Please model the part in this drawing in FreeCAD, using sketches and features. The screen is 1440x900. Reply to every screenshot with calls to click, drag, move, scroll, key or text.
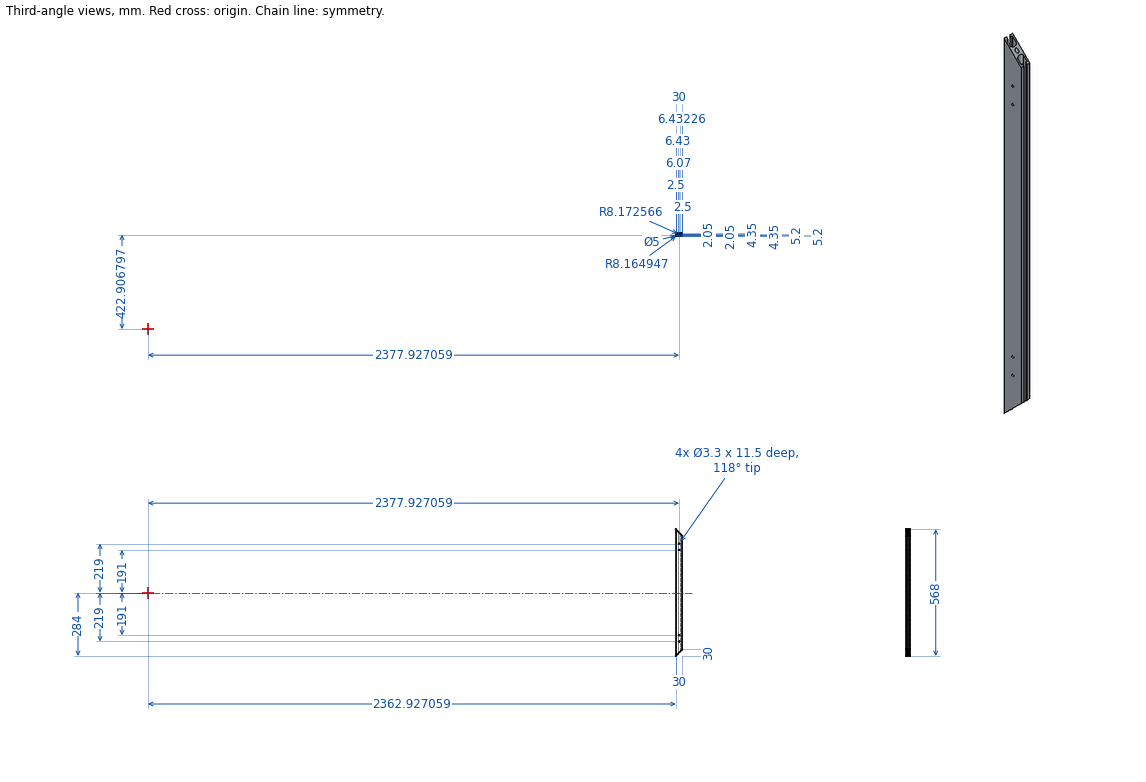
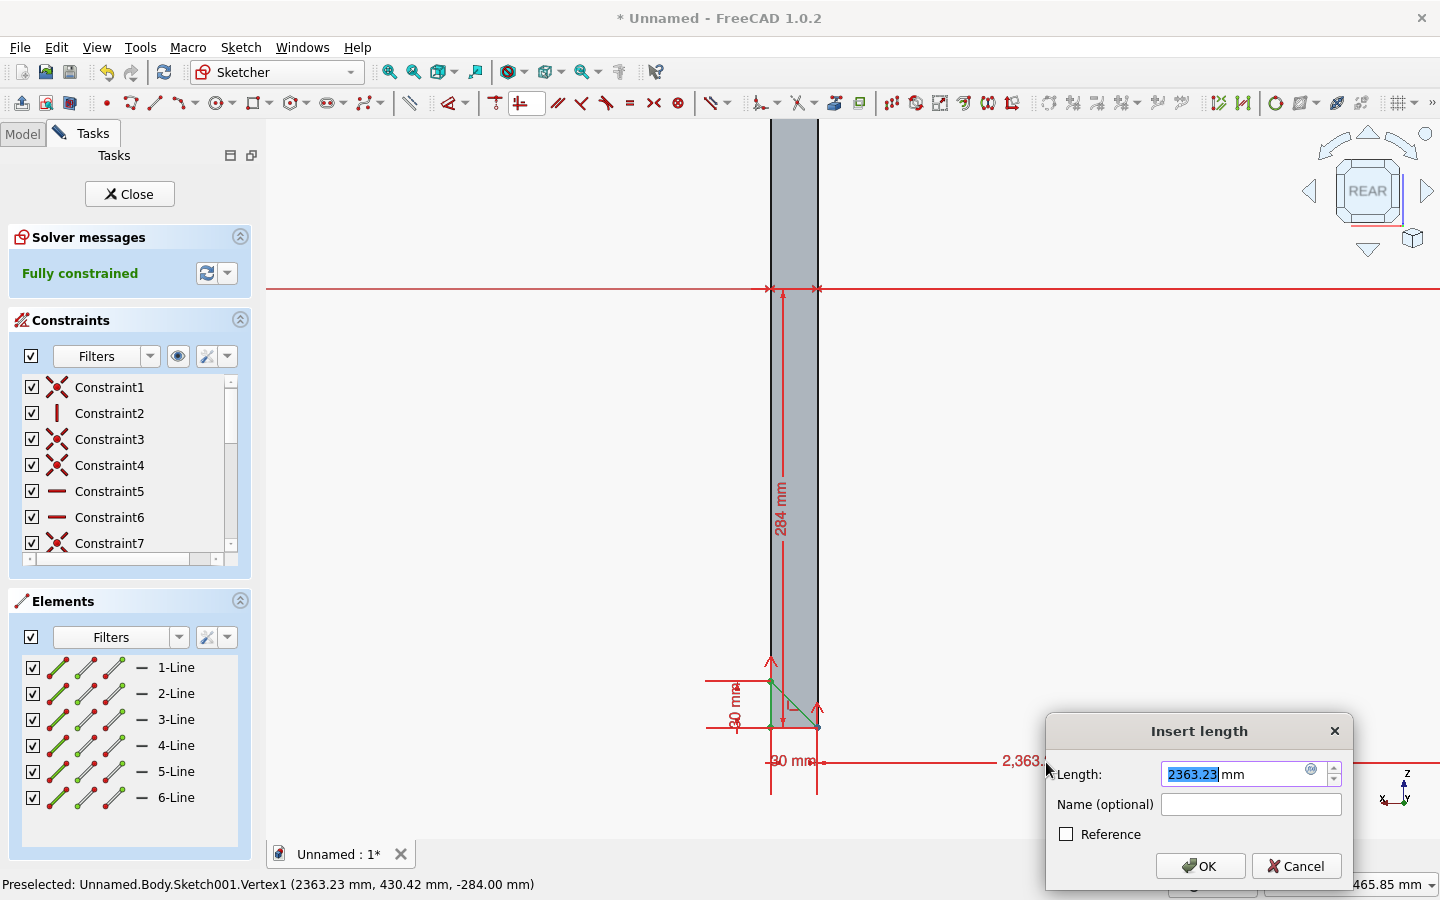
text(2362.927059)
key(Return)
key(Escape)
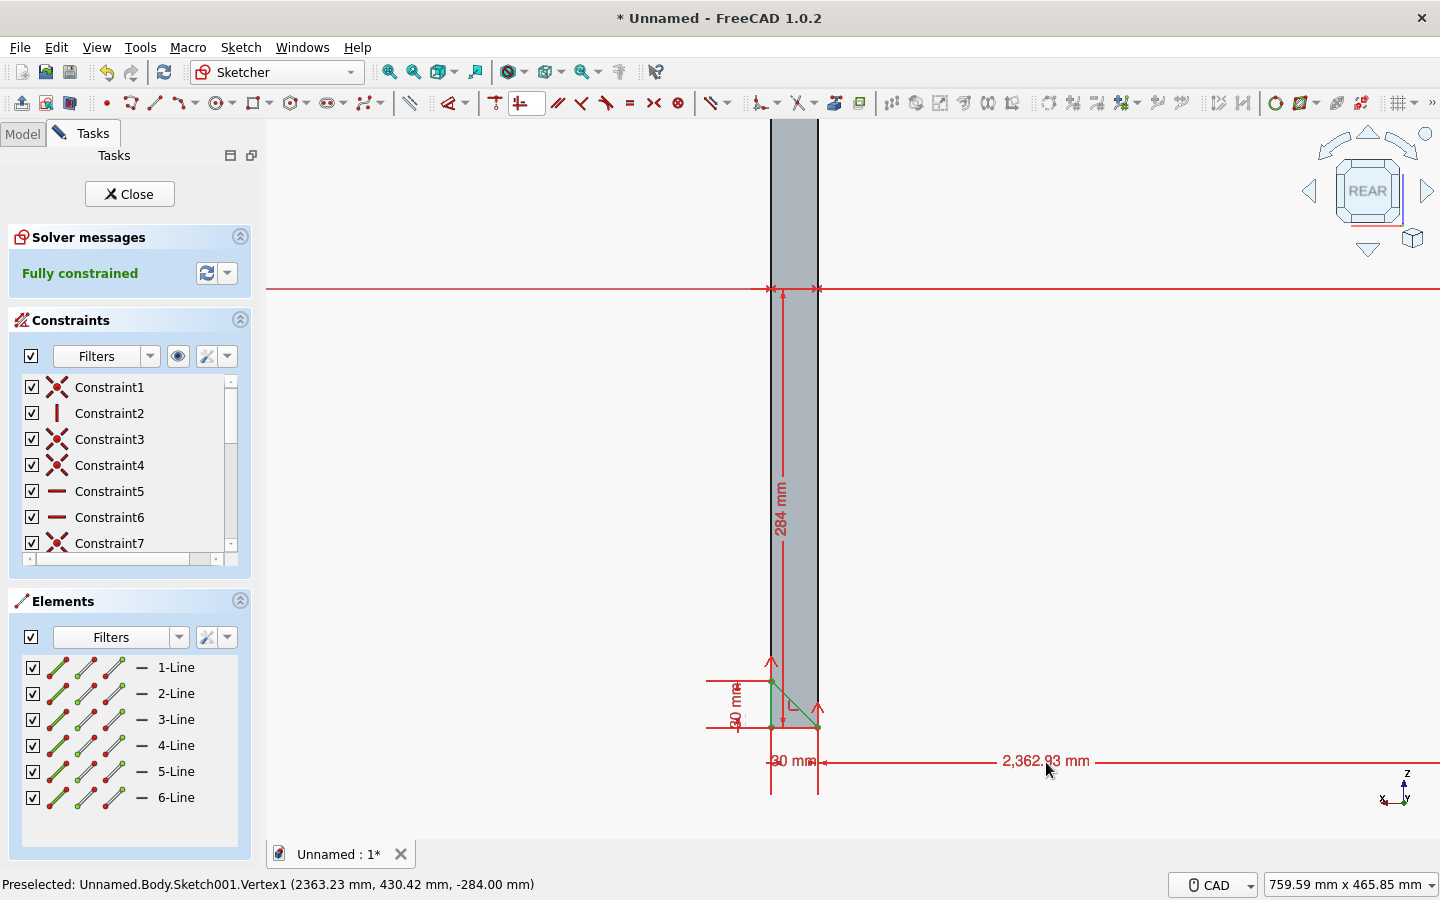
click(130, 194)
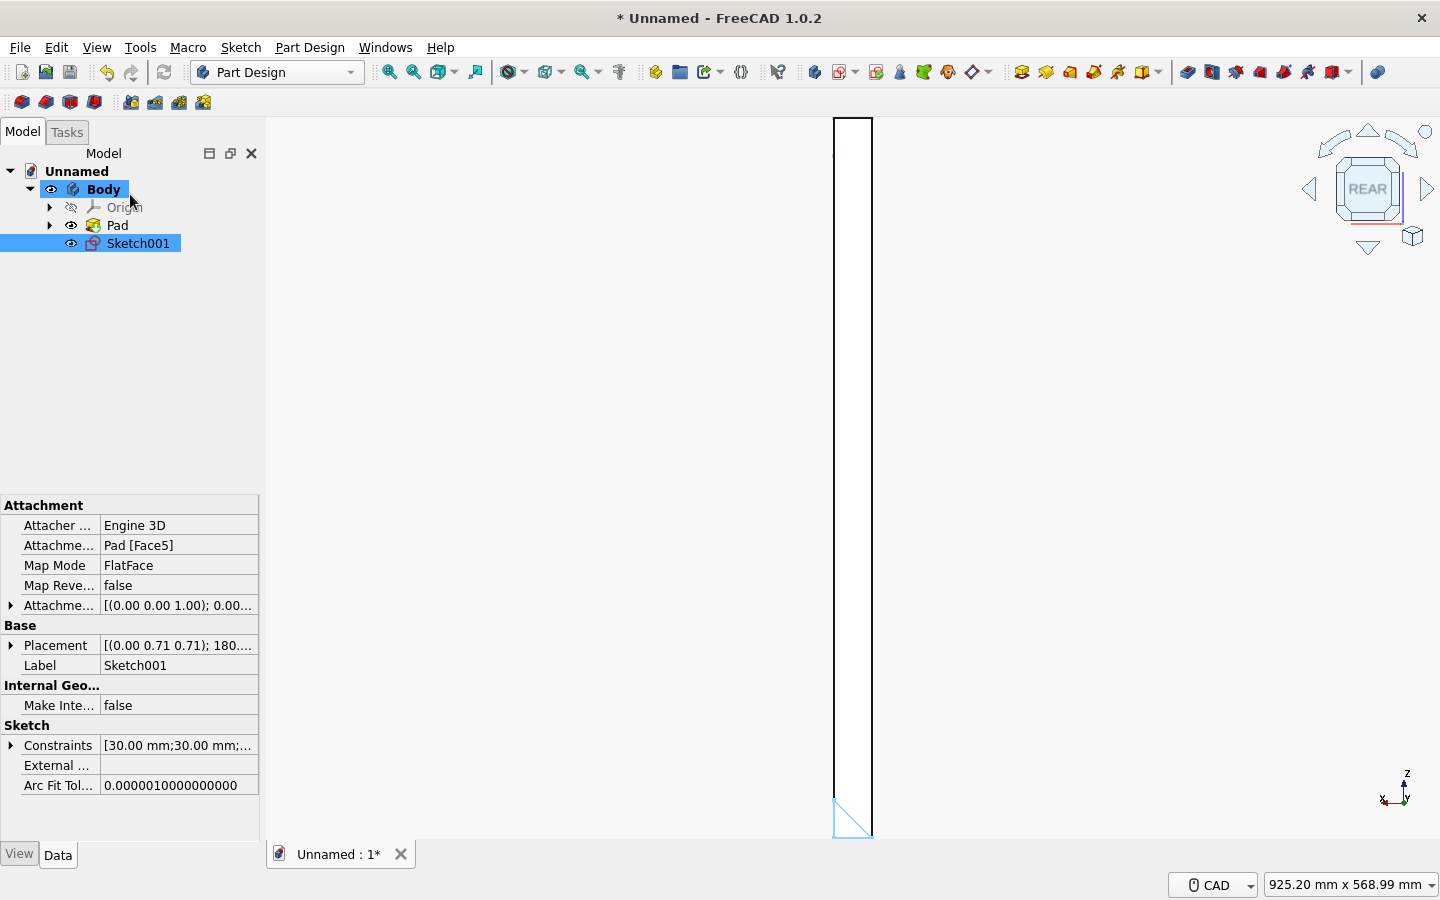
click(1188, 72)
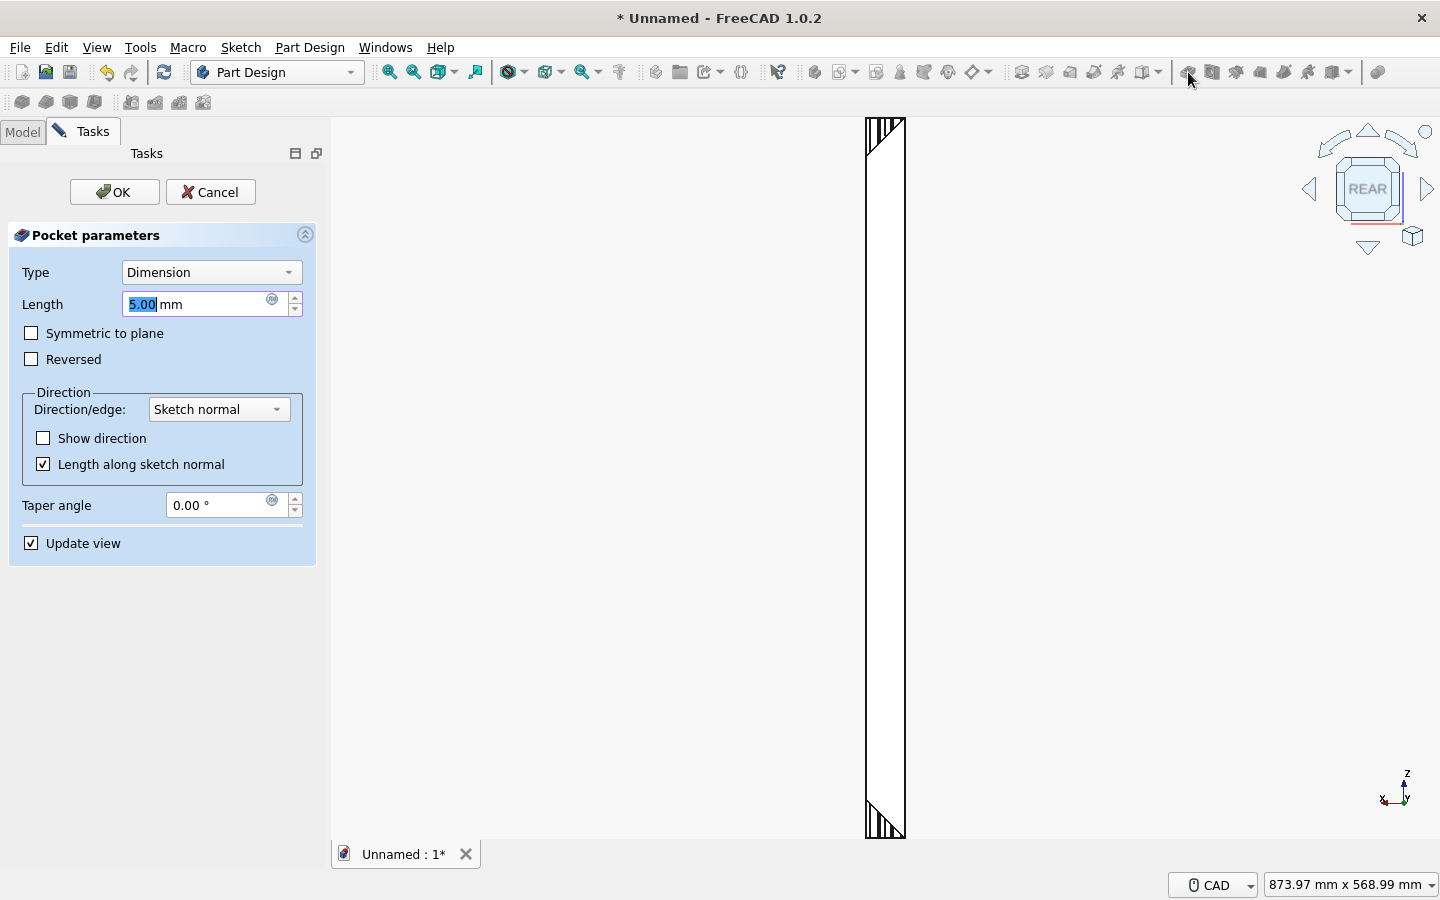
click(212, 272)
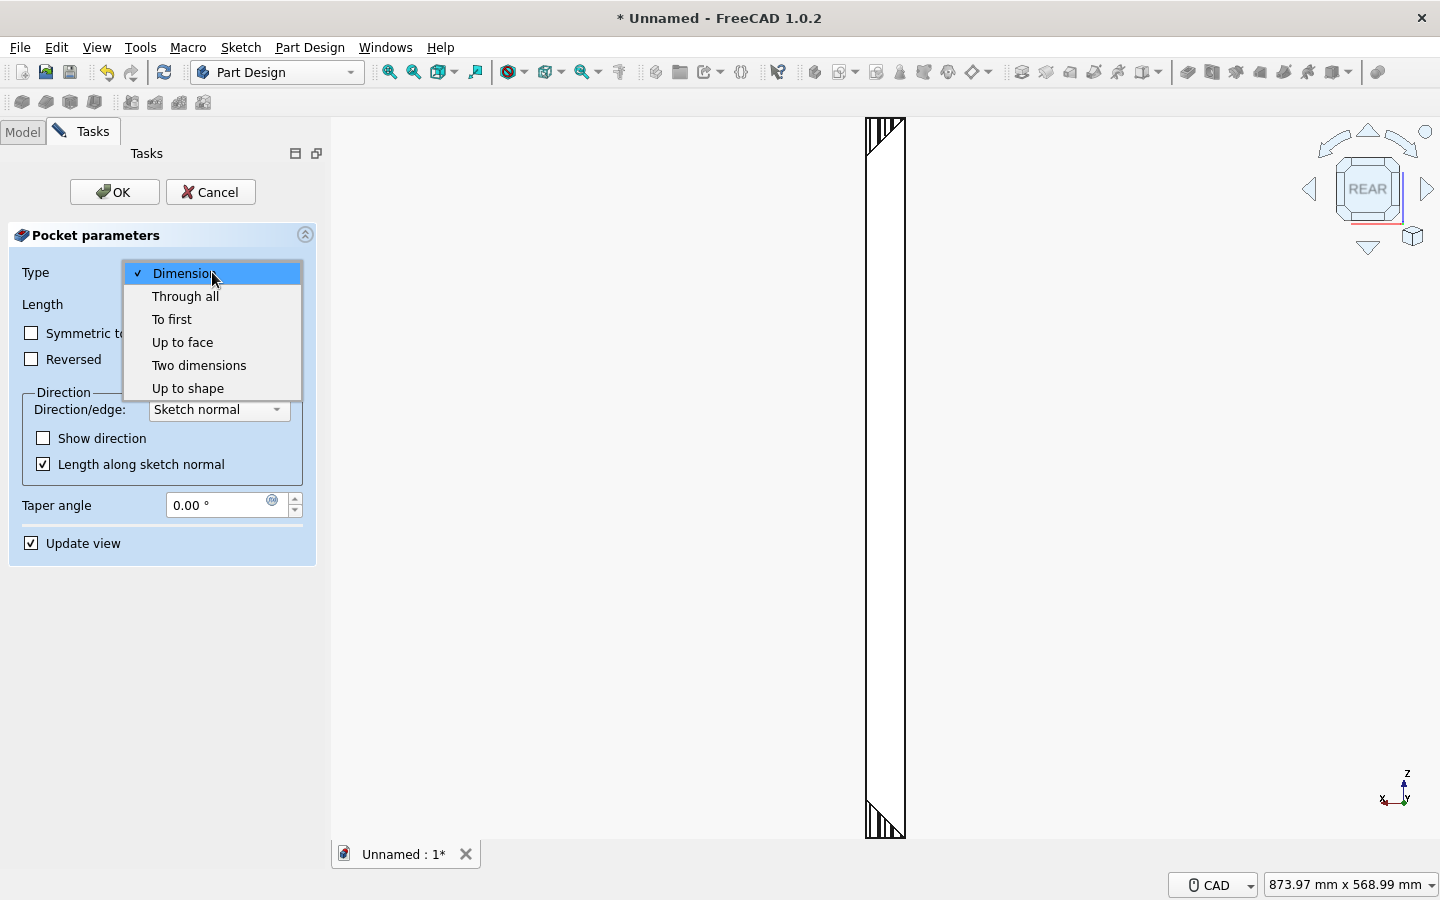
click(212, 296)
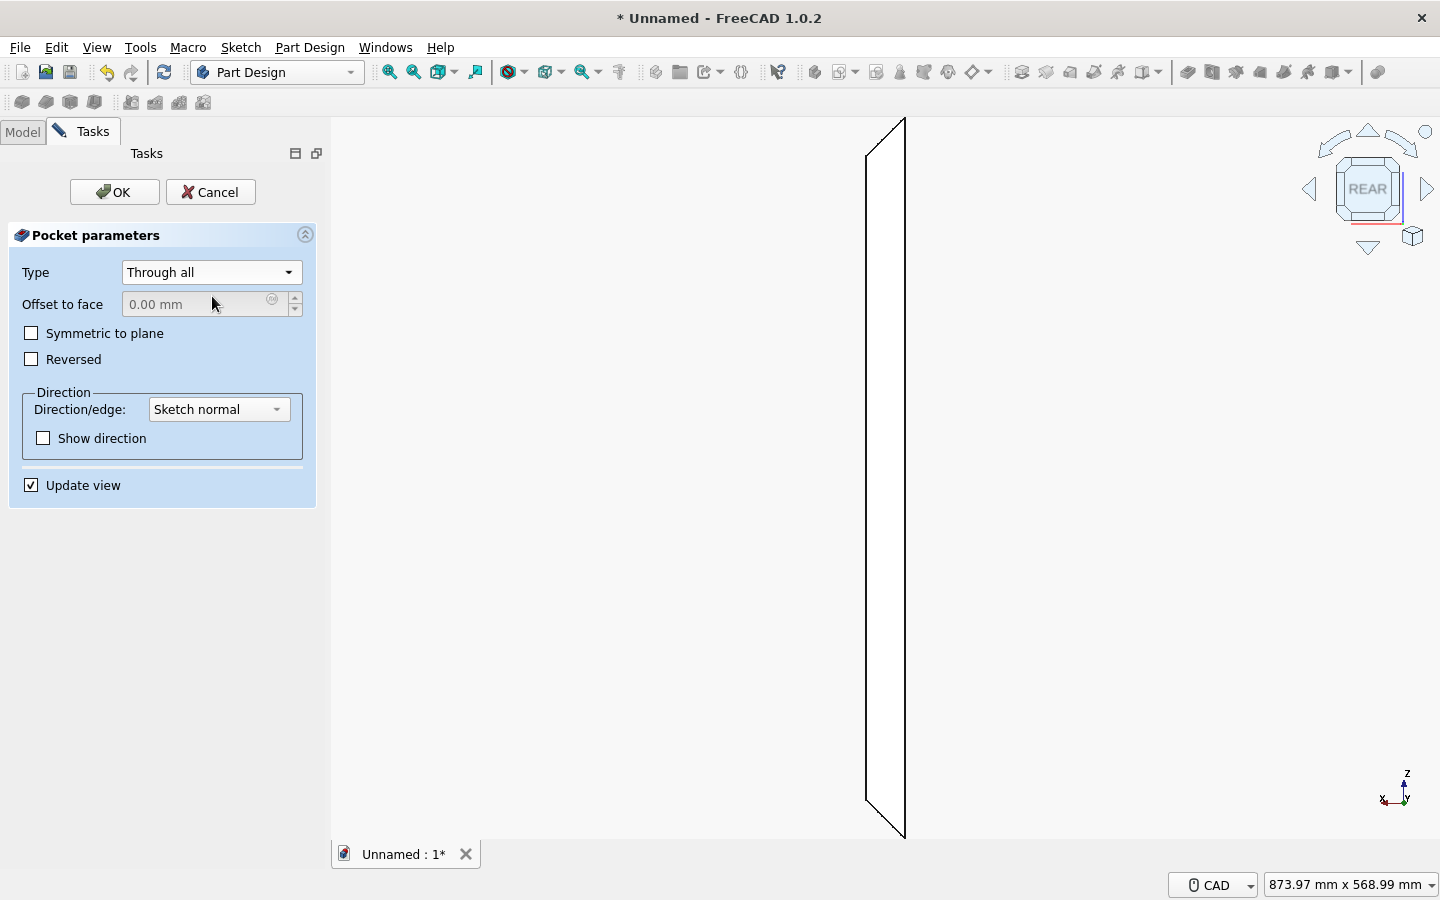
click(115, 192)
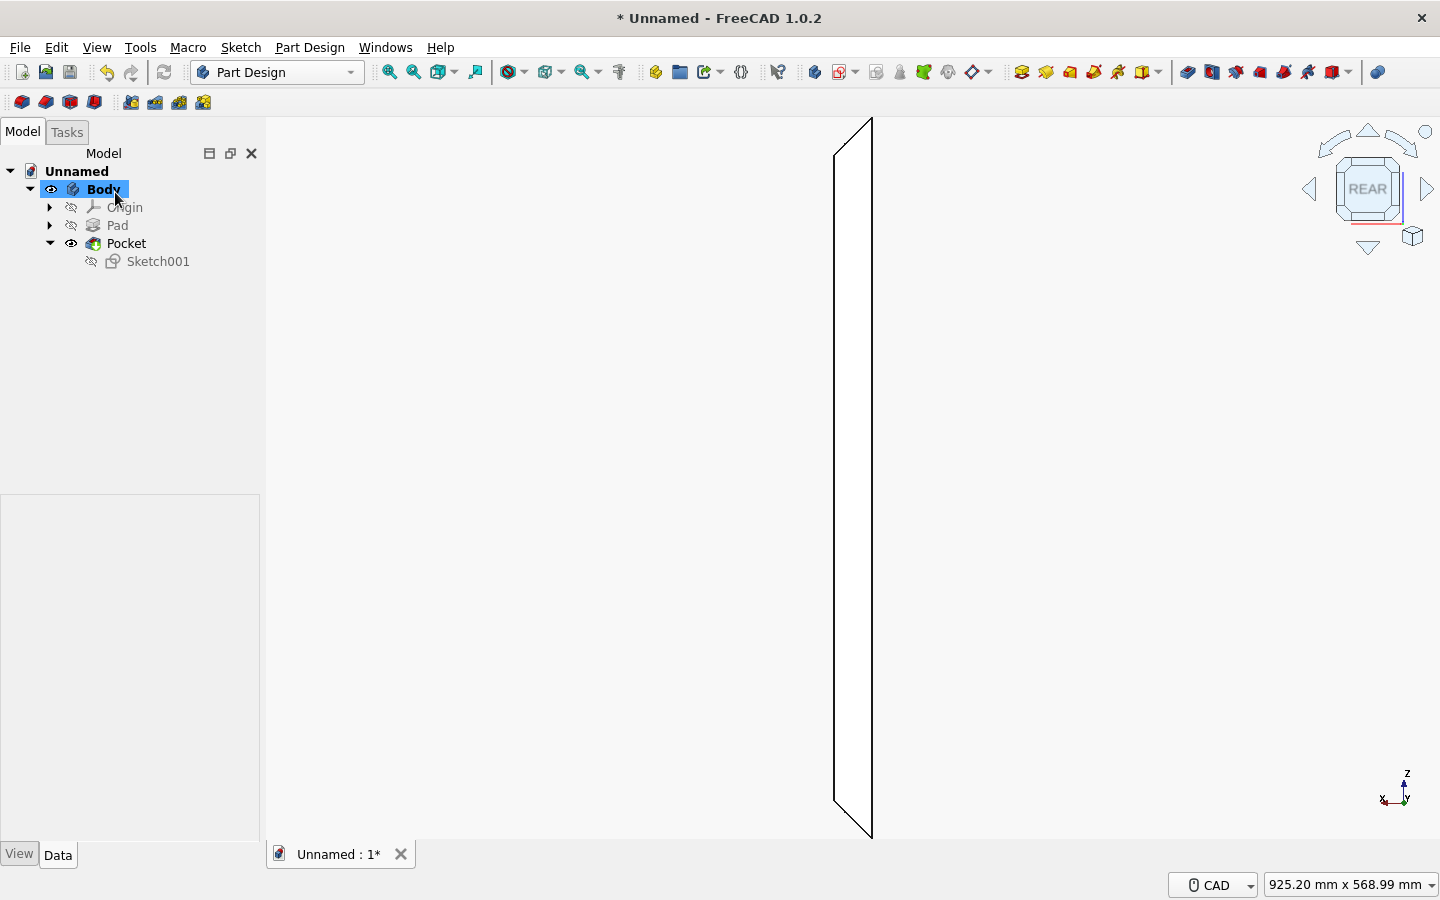
key(0)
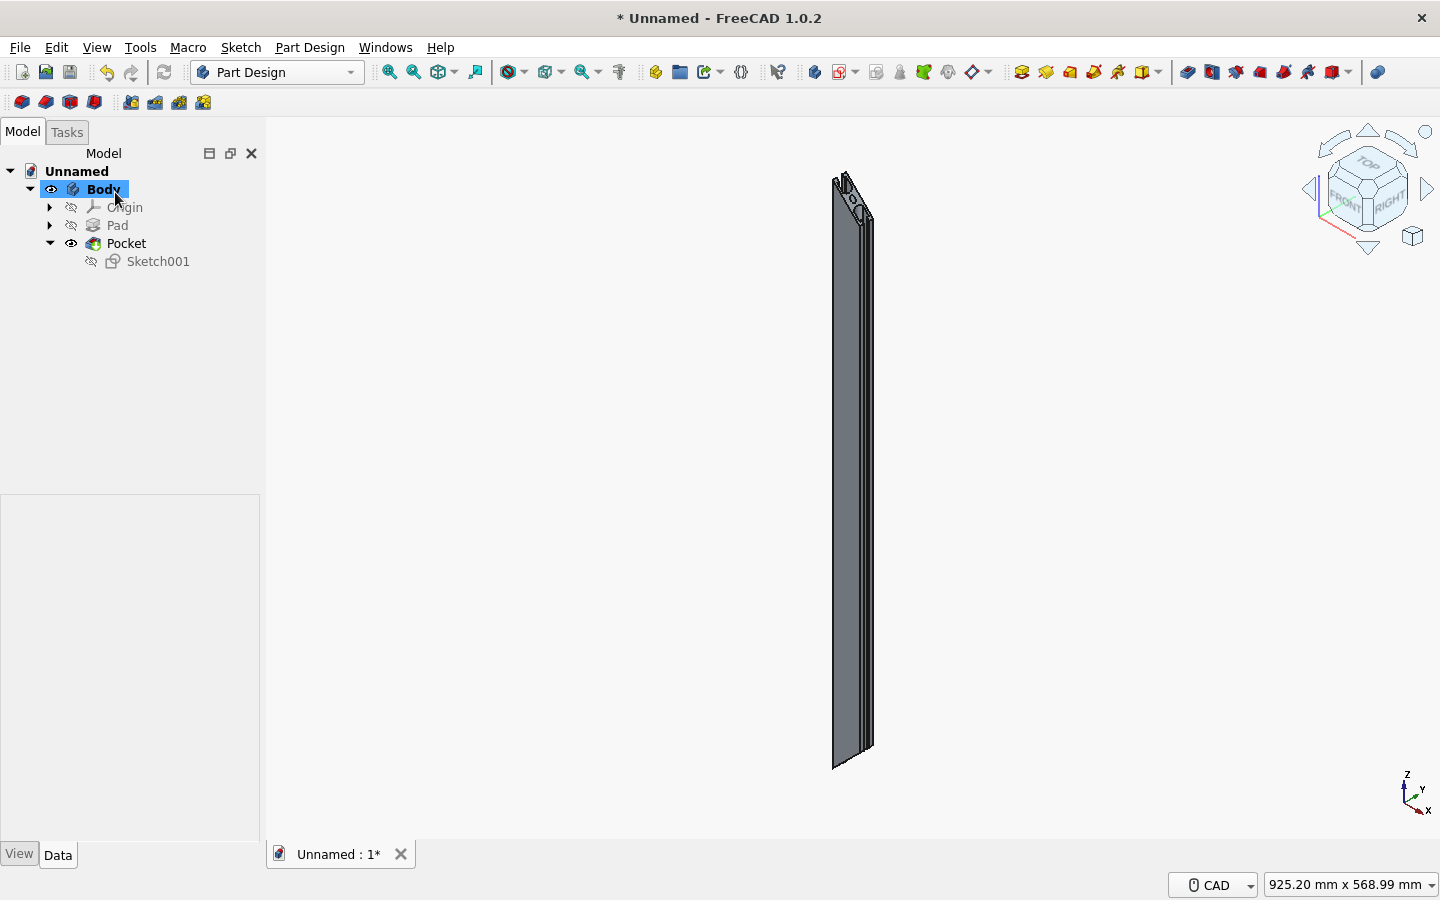
click(850, 231)